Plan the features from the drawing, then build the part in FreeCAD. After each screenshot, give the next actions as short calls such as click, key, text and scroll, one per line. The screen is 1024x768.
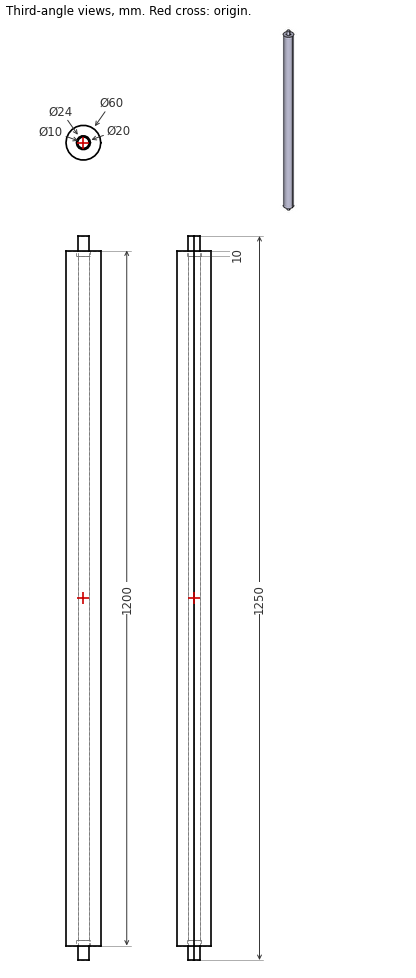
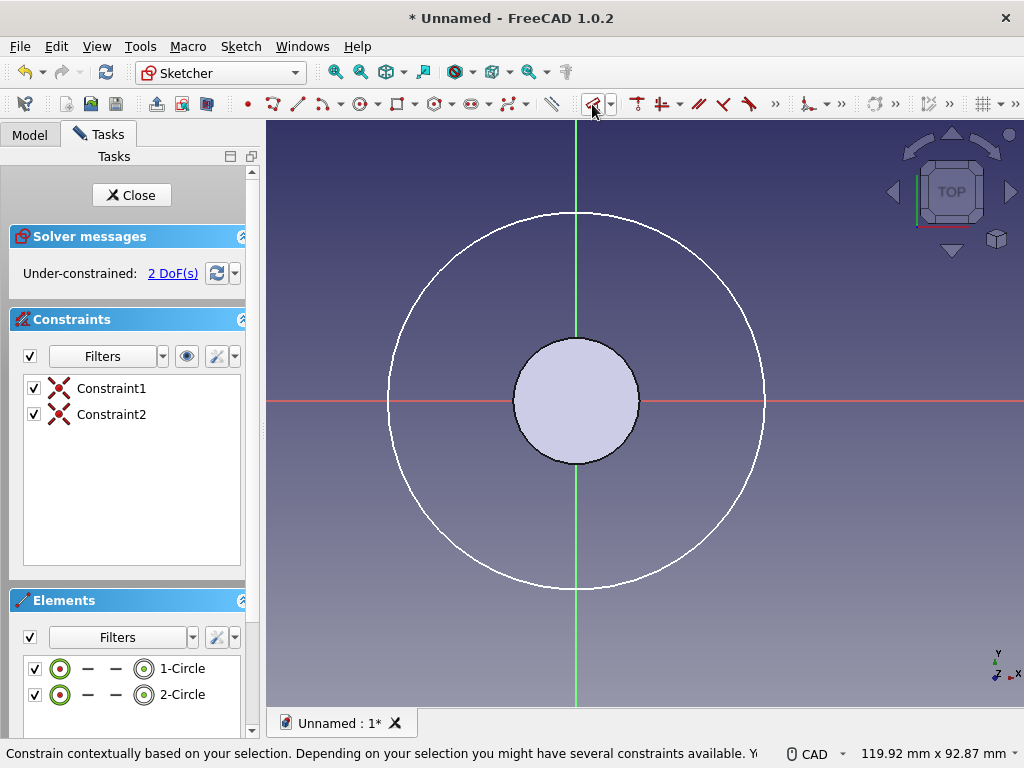
click(709, 267)
click(732, 244)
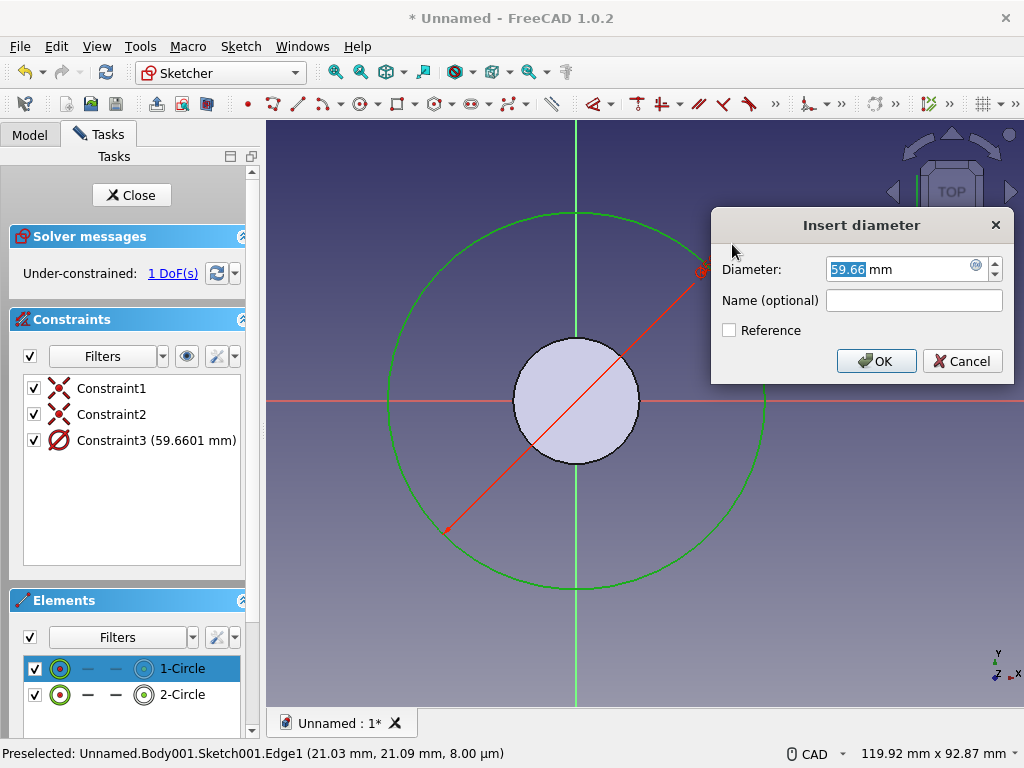
text(60)
key(Return)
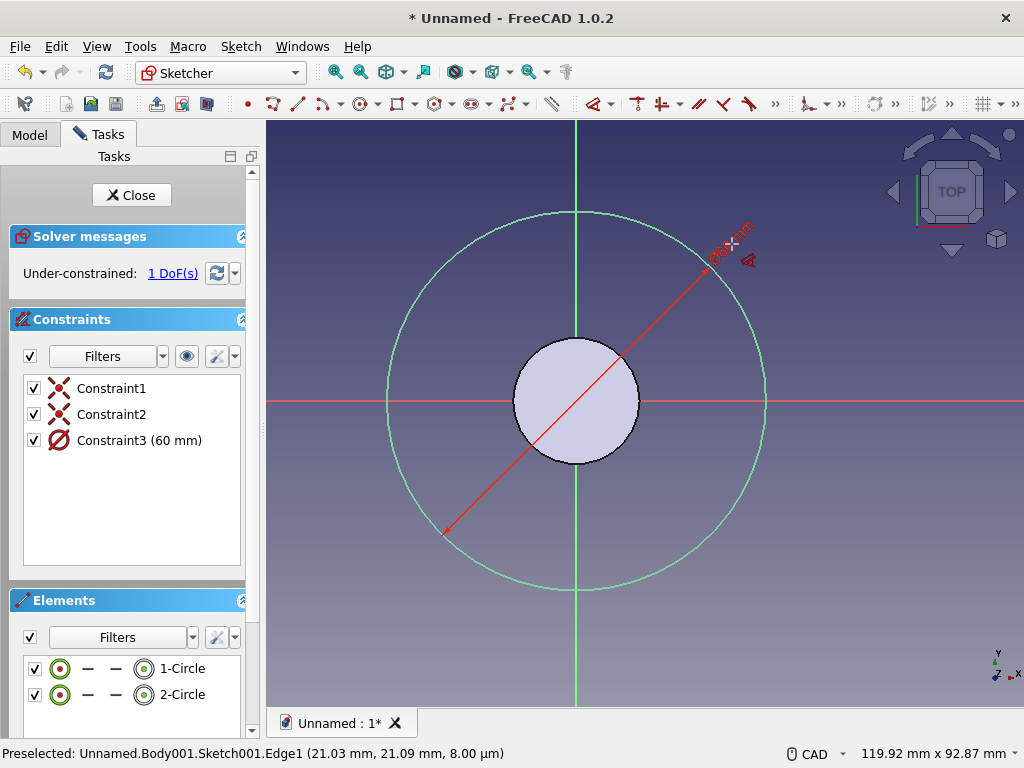
click(621, 357)
click(644, 335)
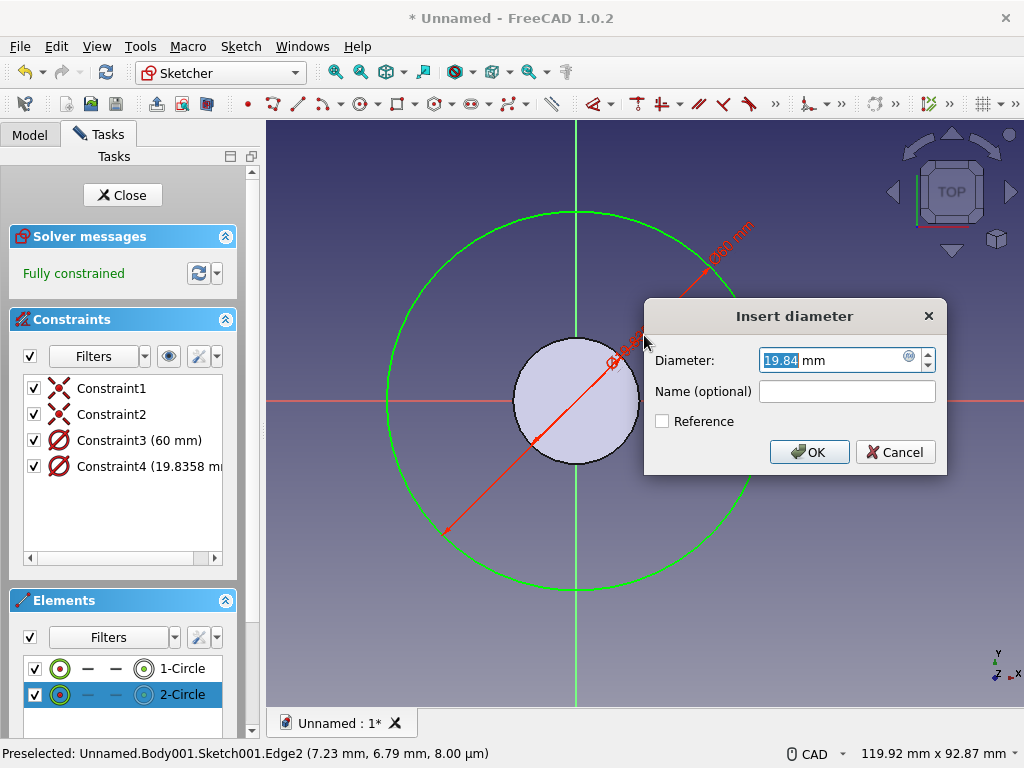
text(20)
key(Return)
key(Escape)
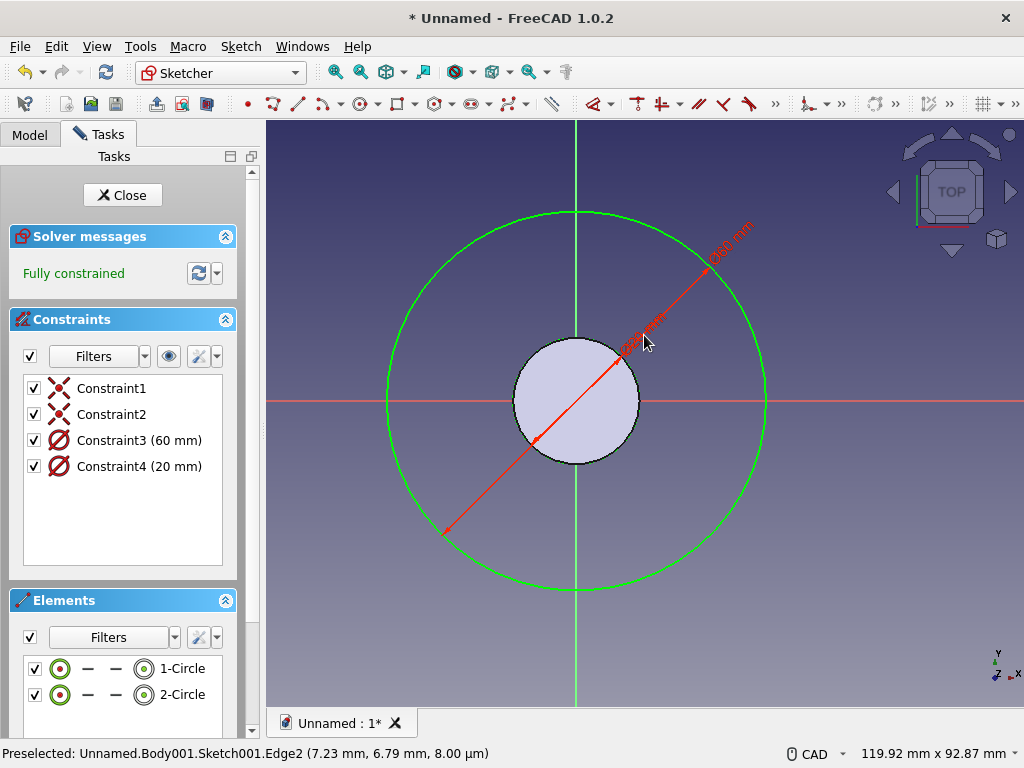
click(123, 195)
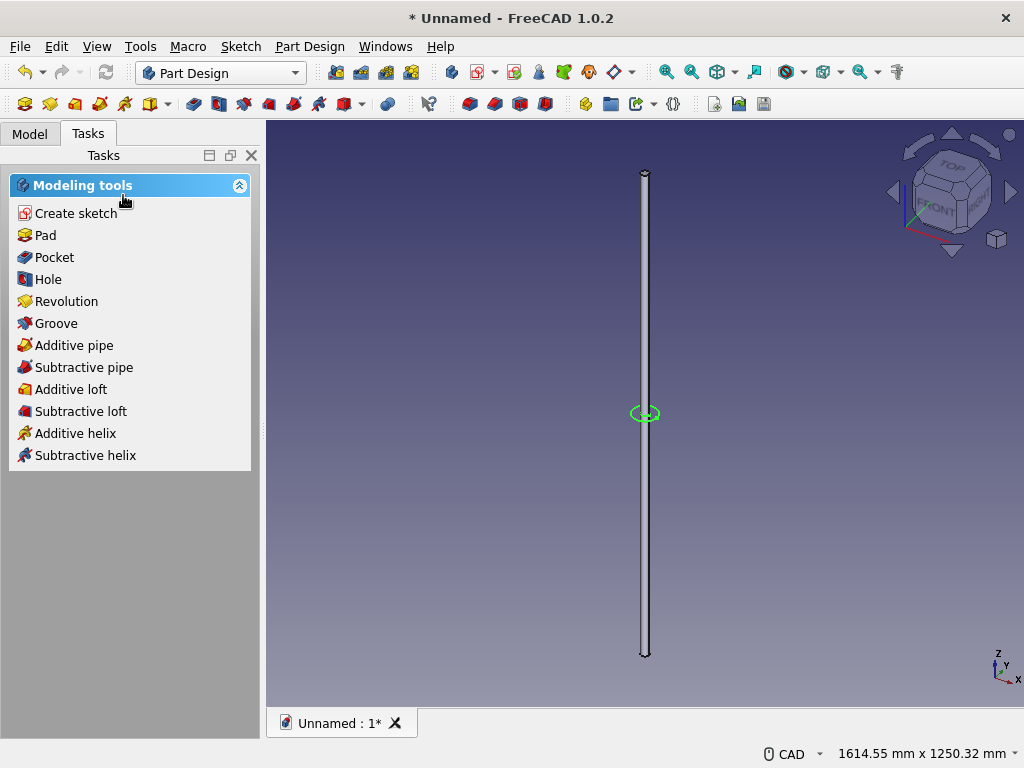
click(25, 104)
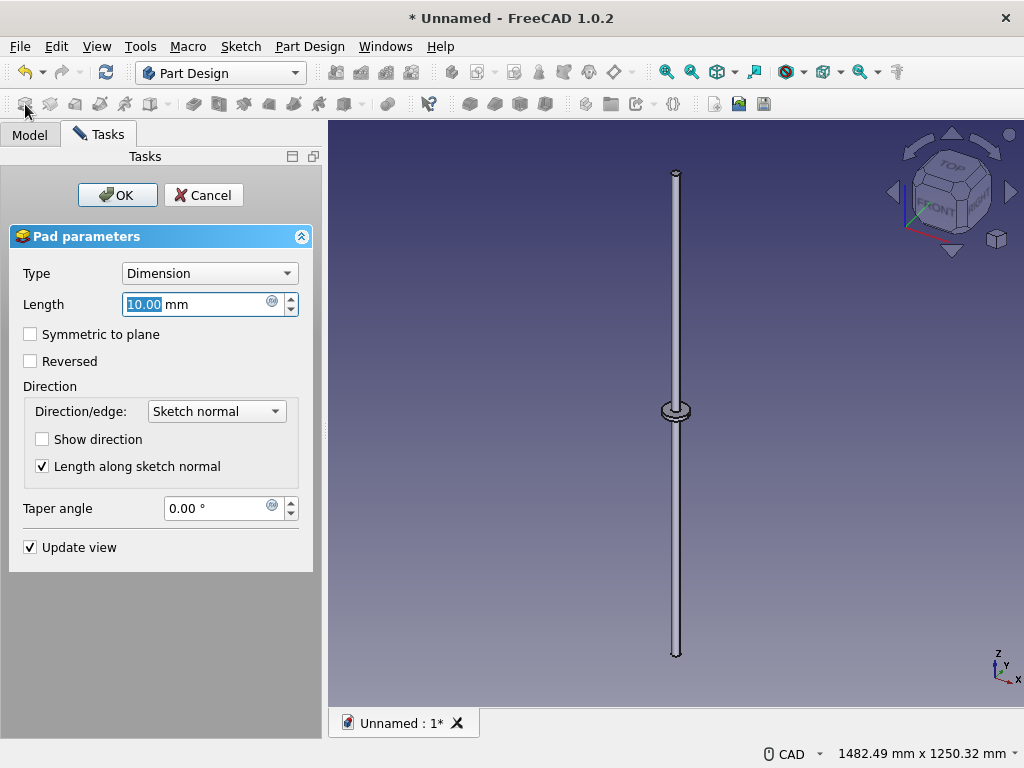
text(1200)
key(Tab)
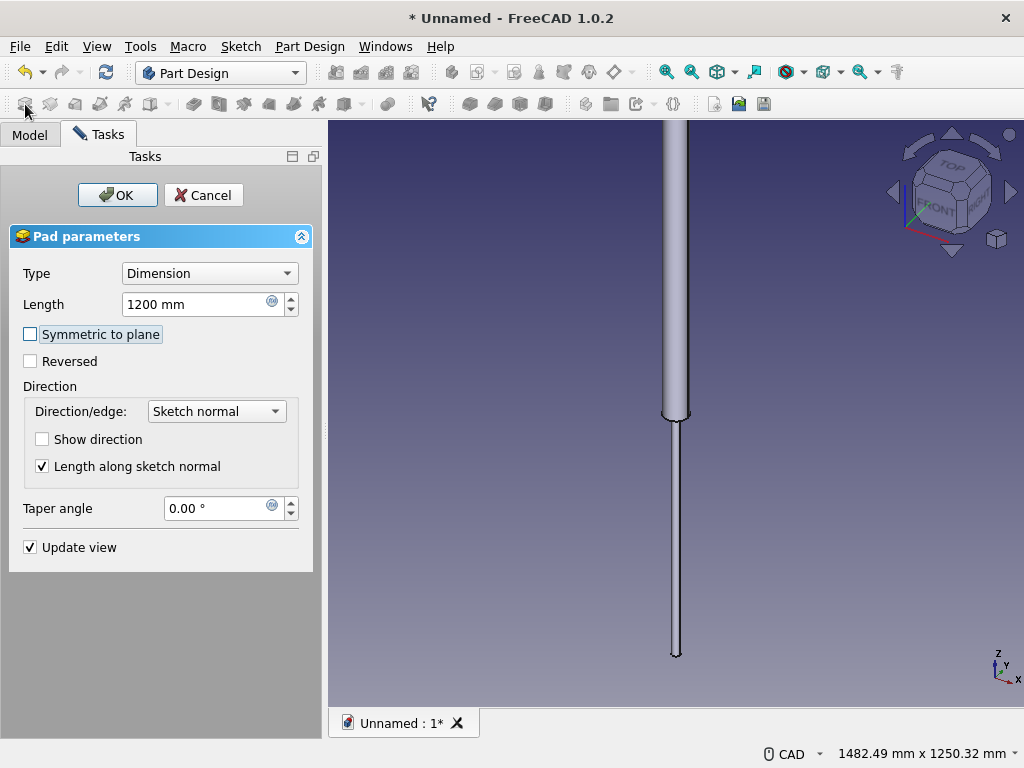
click(31, 334)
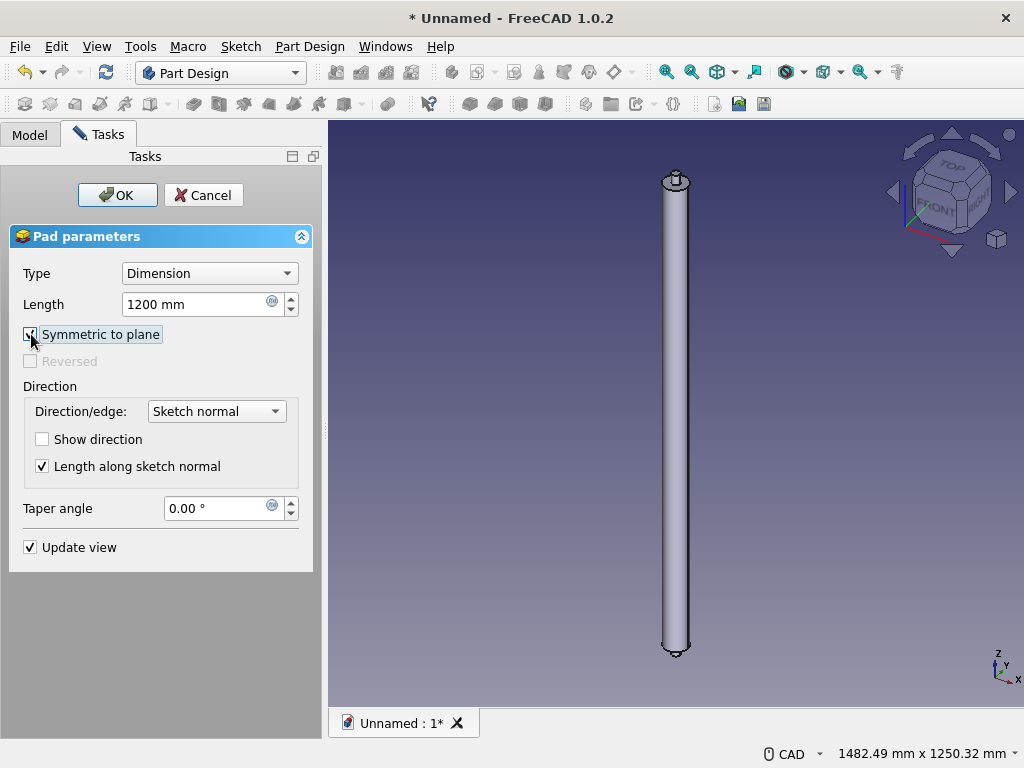
click(118, 195)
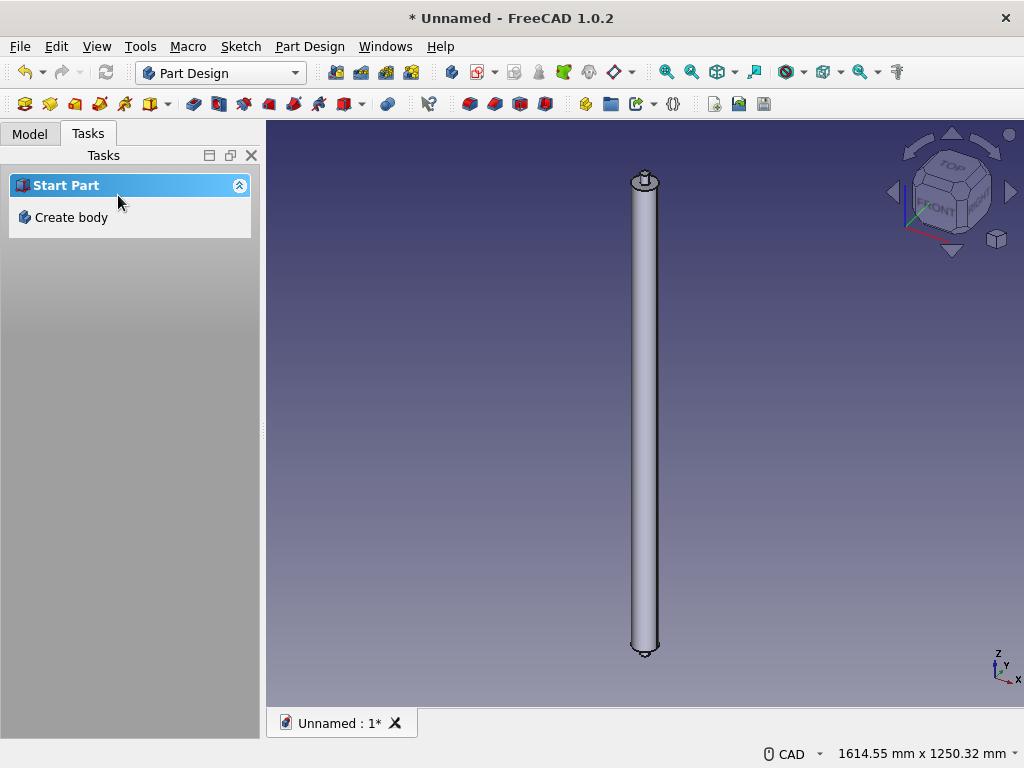
scroll(646, 177, up, 6)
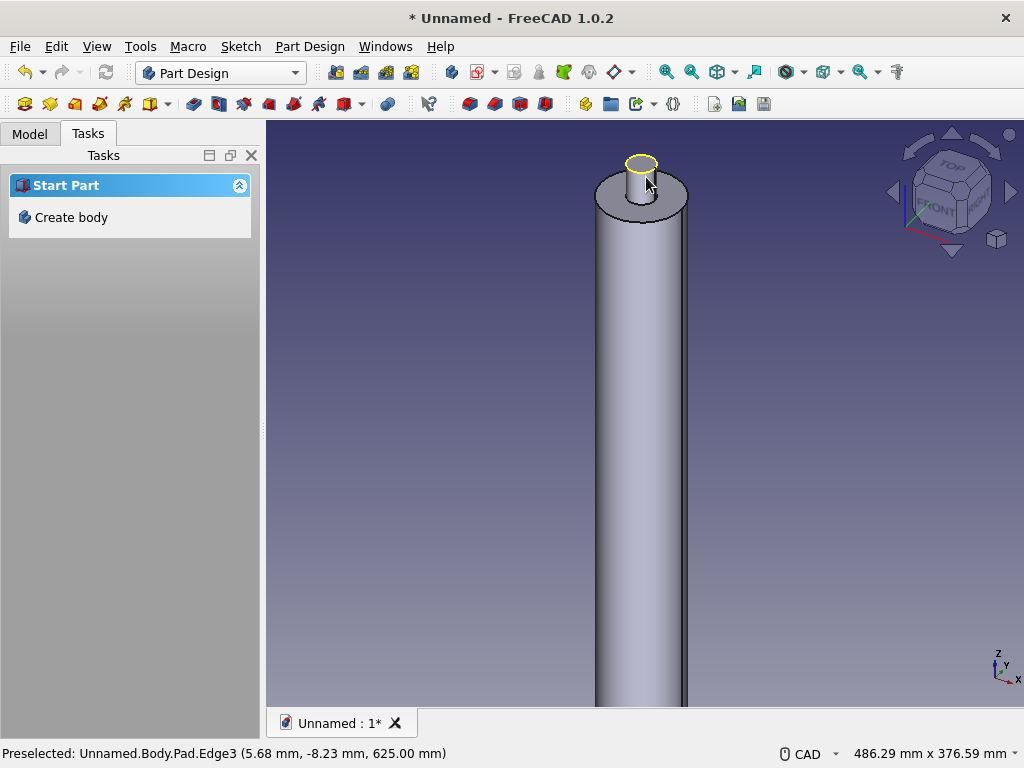
click(671, 196)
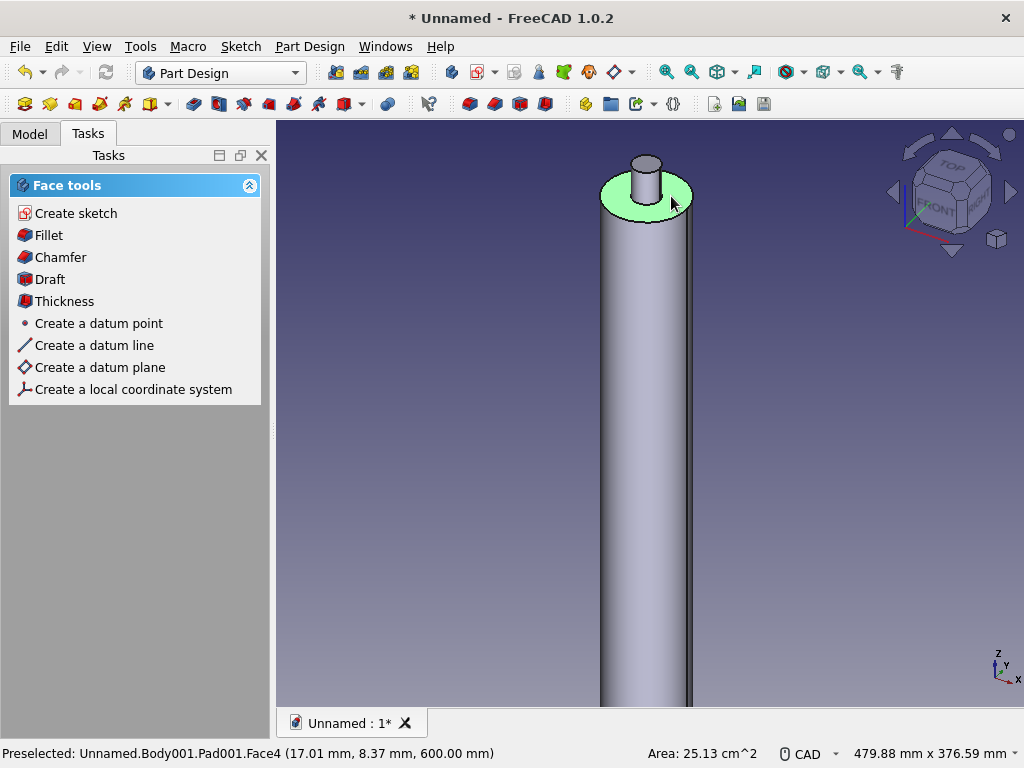
click(476, 72)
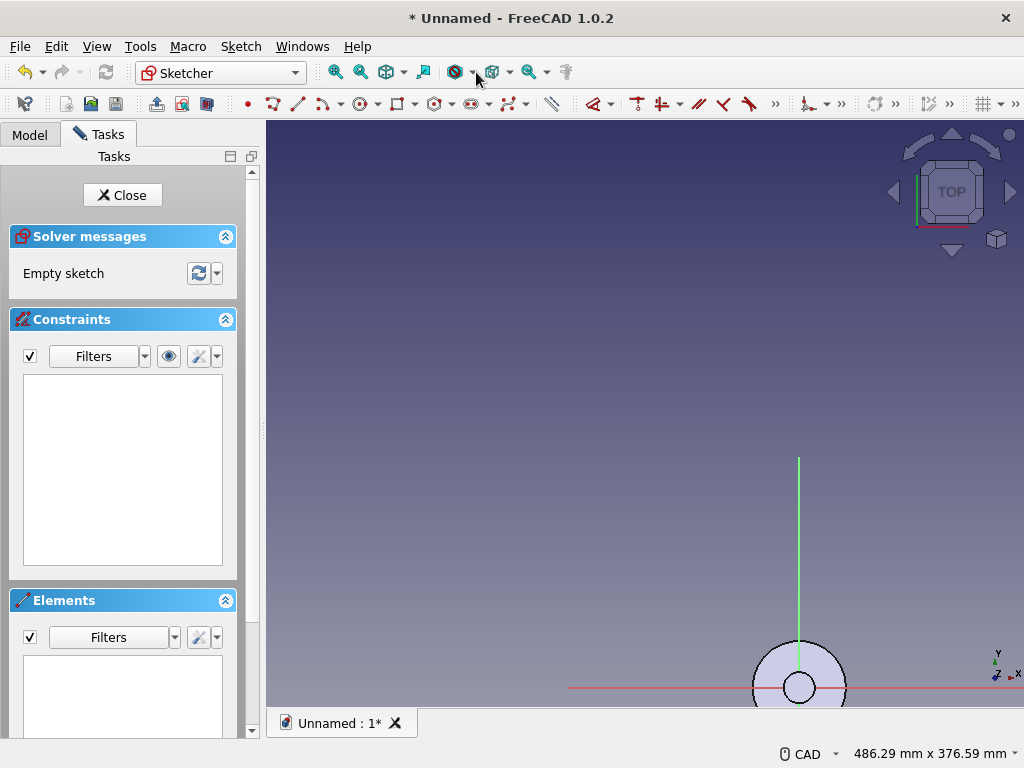
scroll(576, 414, down, 5)